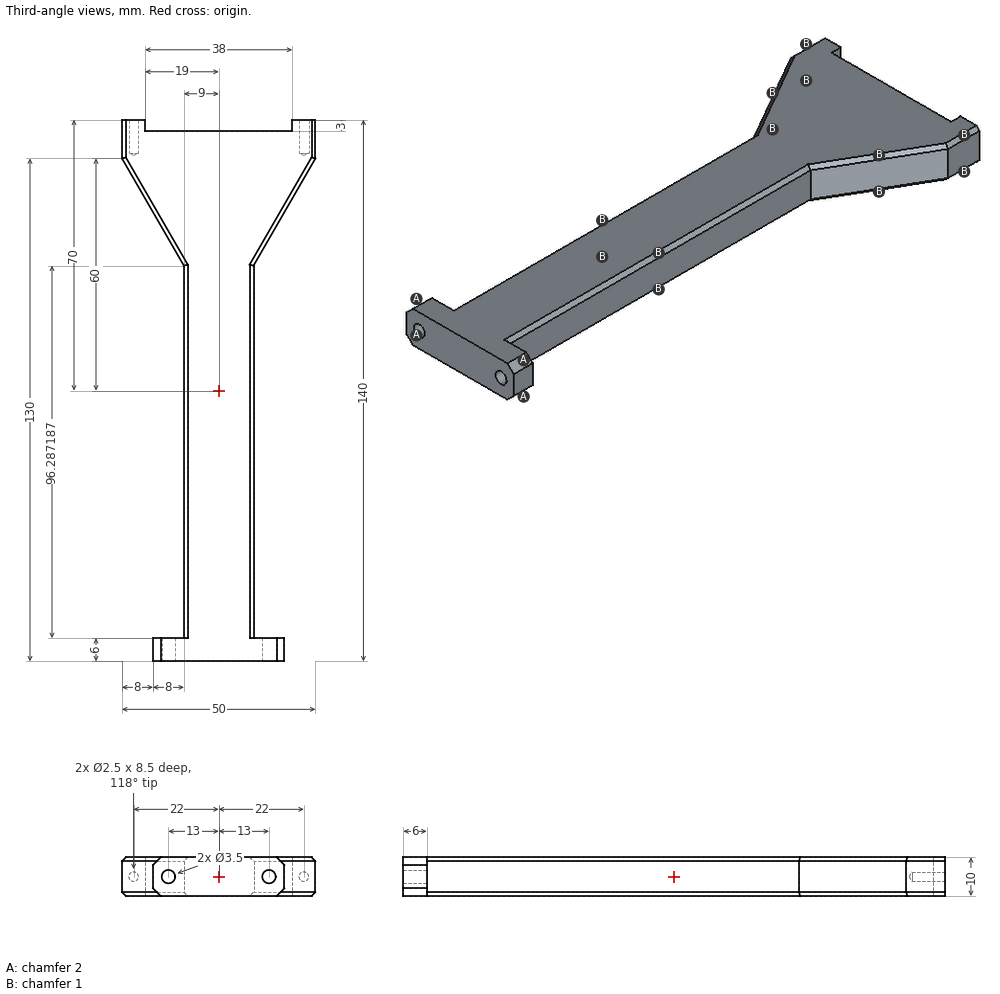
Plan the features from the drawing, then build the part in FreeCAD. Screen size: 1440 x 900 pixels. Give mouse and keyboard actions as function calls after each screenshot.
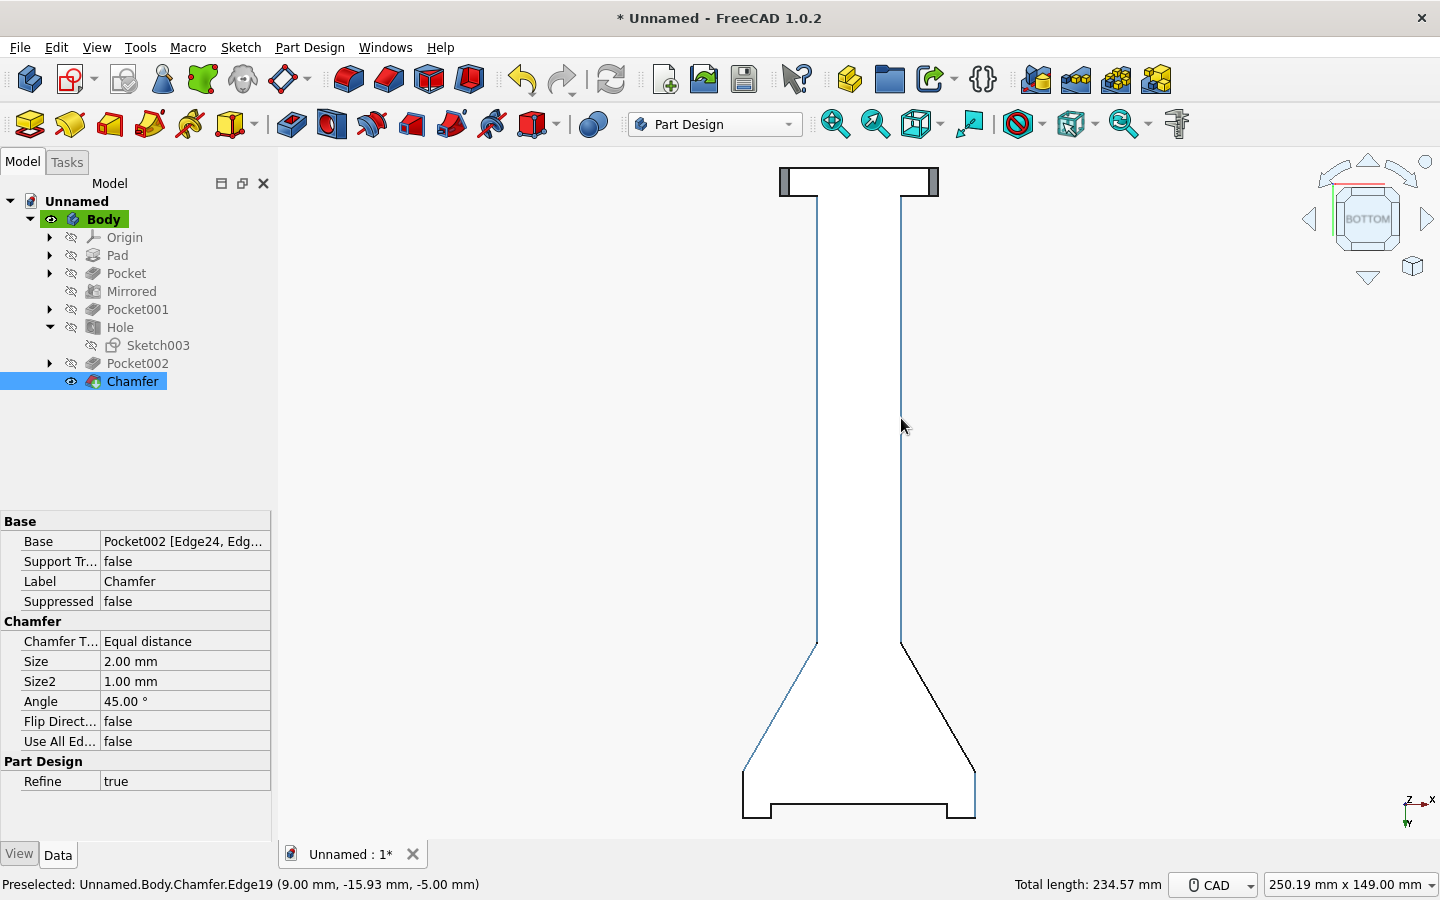
click(938, 706, ctrl)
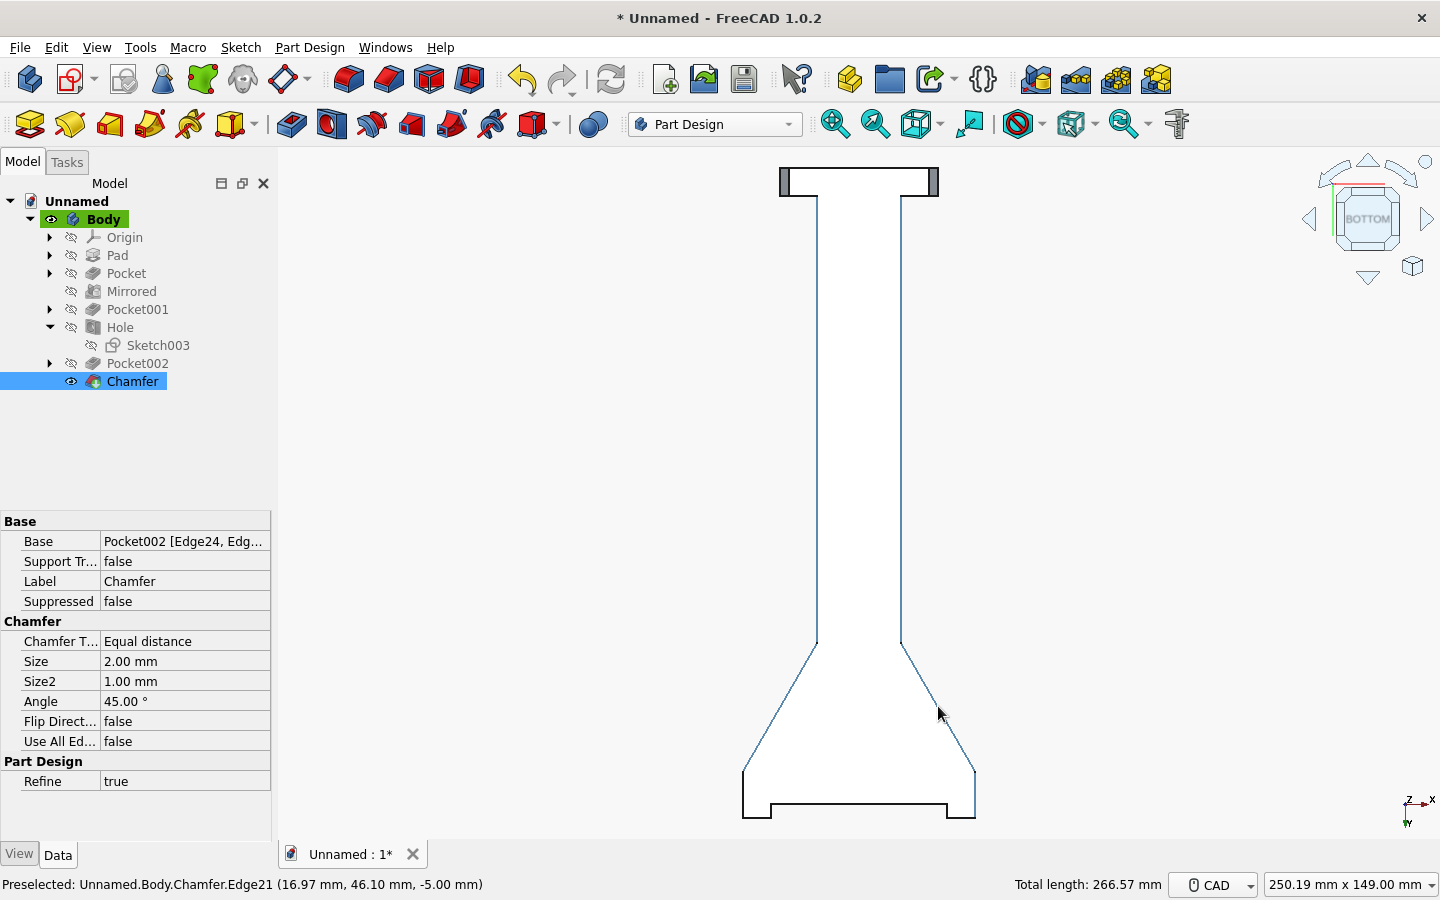
click(743, 794, ctrl)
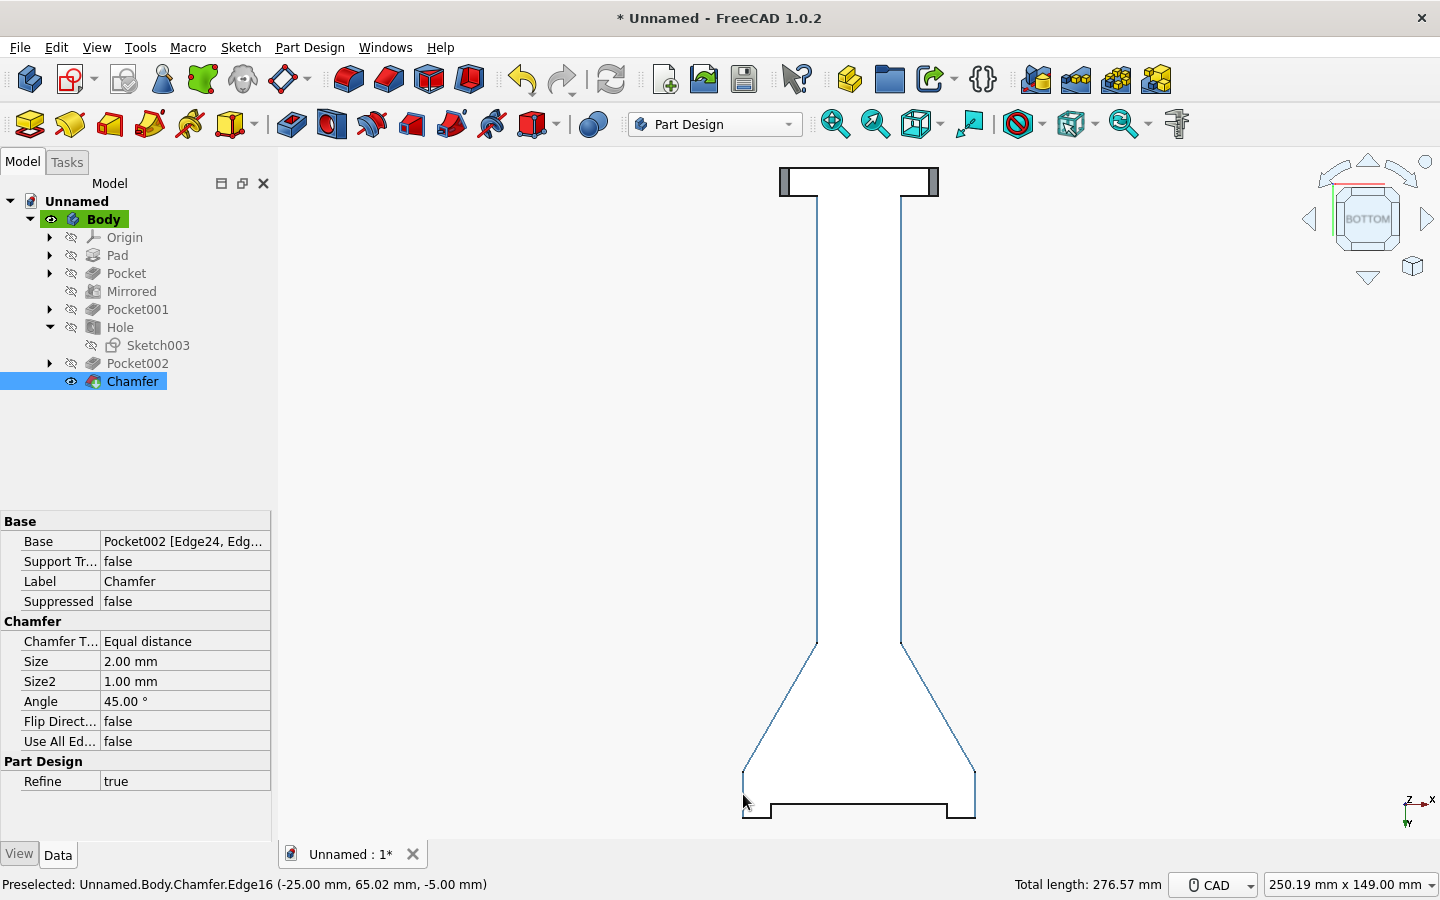
key(0)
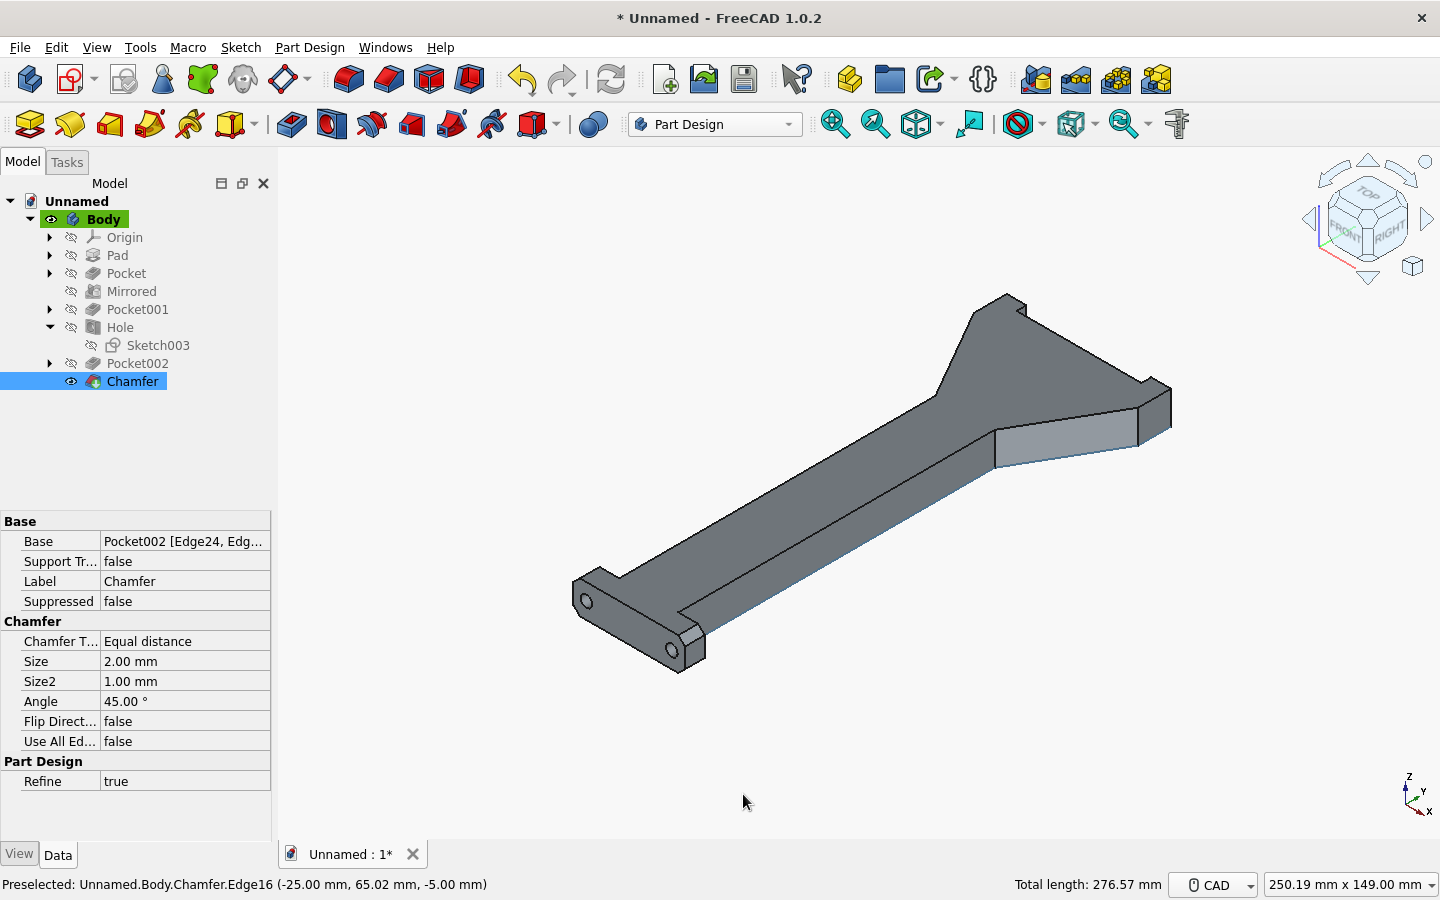
click(1155, 397, ctrl)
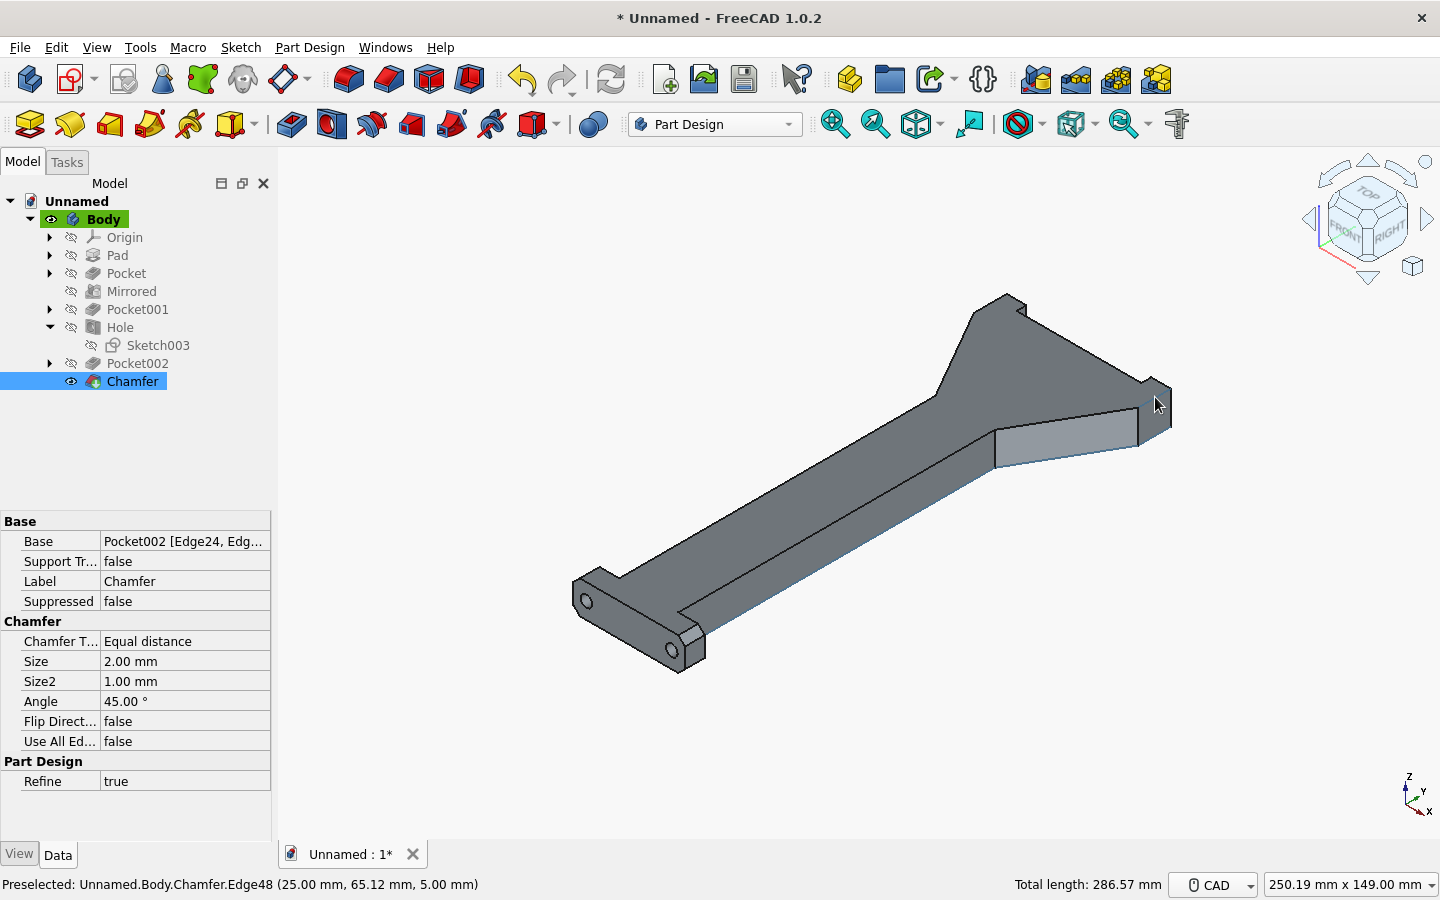
click(836, 520, ctrl)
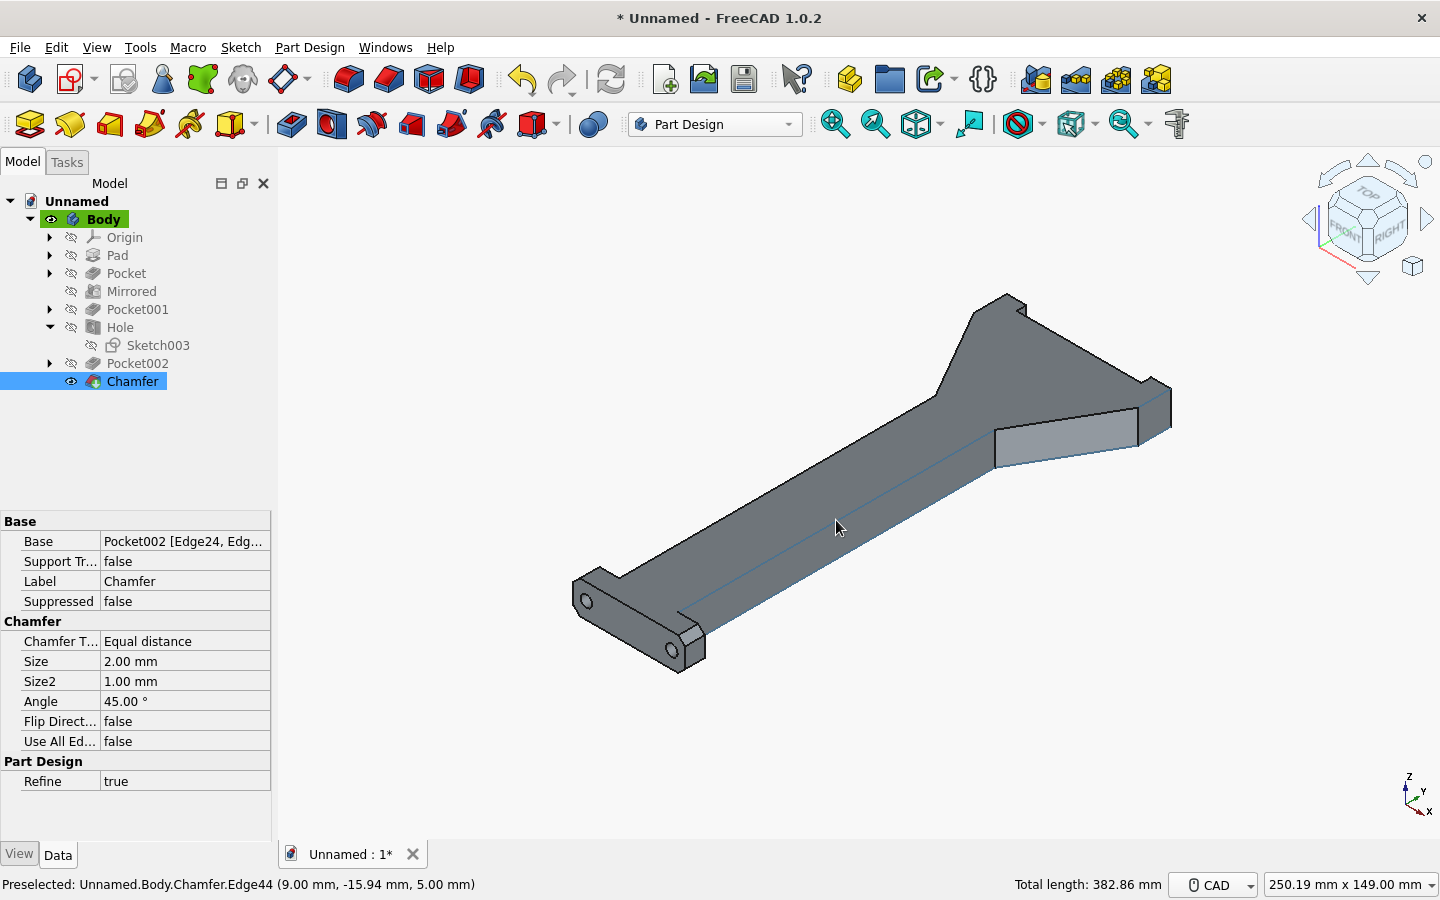
click(1066, 418, ctrl)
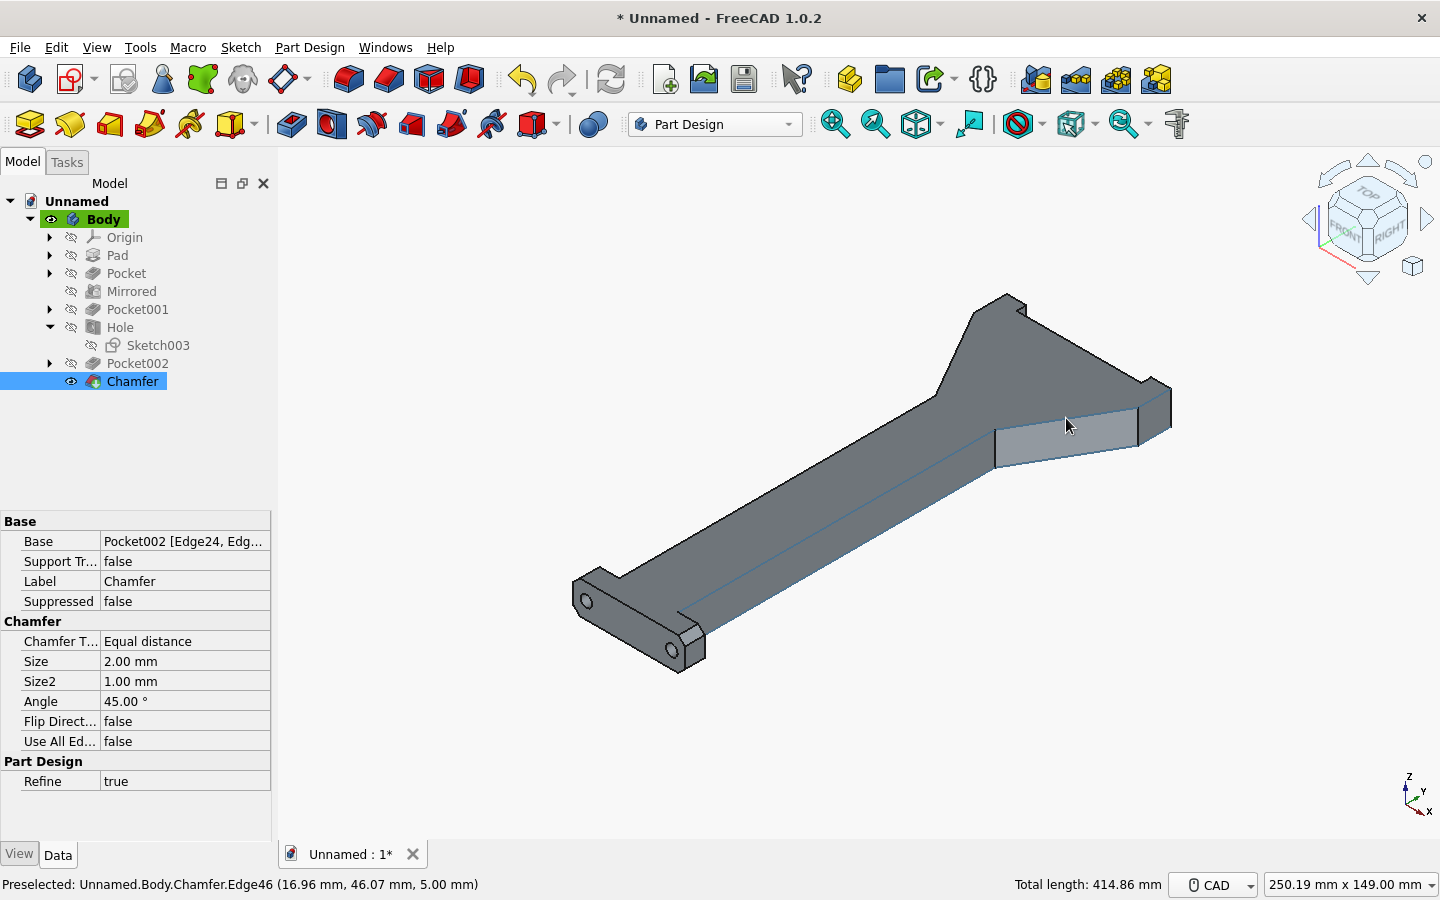
key(2)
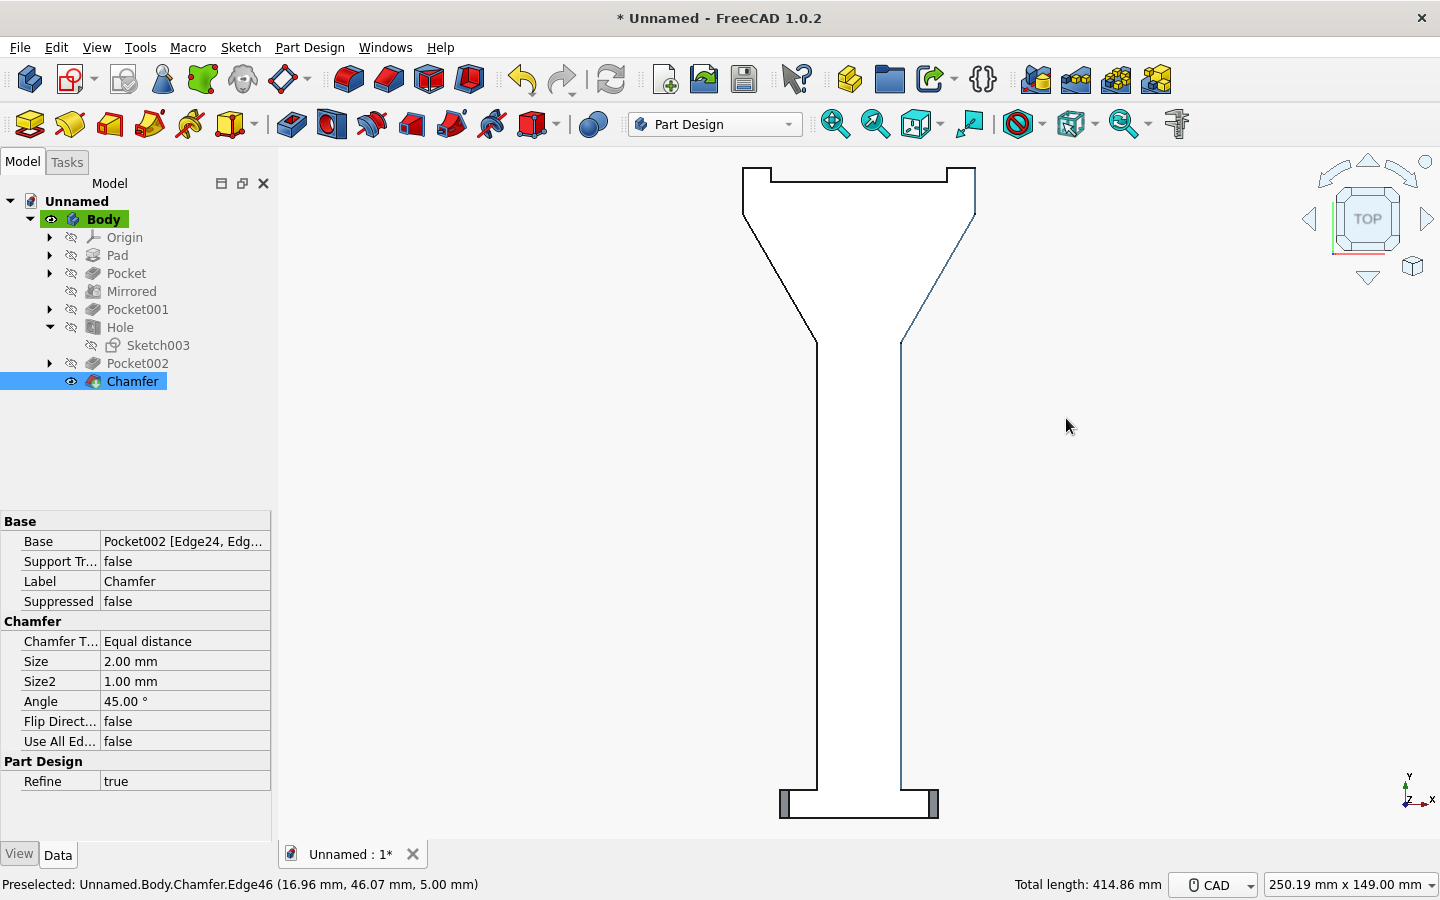
click(743, 190, ctrl)